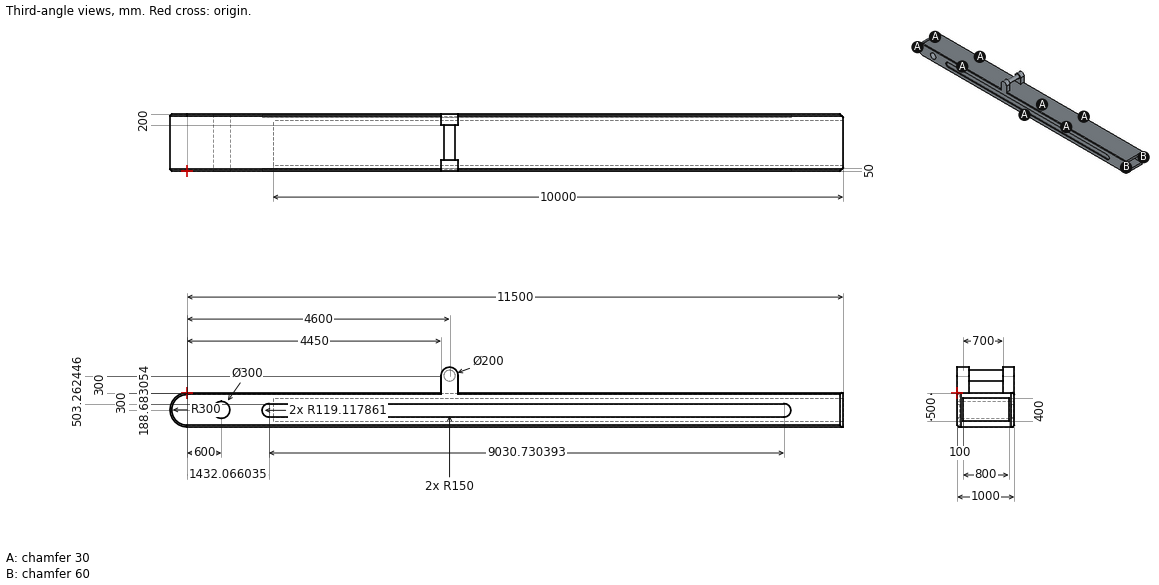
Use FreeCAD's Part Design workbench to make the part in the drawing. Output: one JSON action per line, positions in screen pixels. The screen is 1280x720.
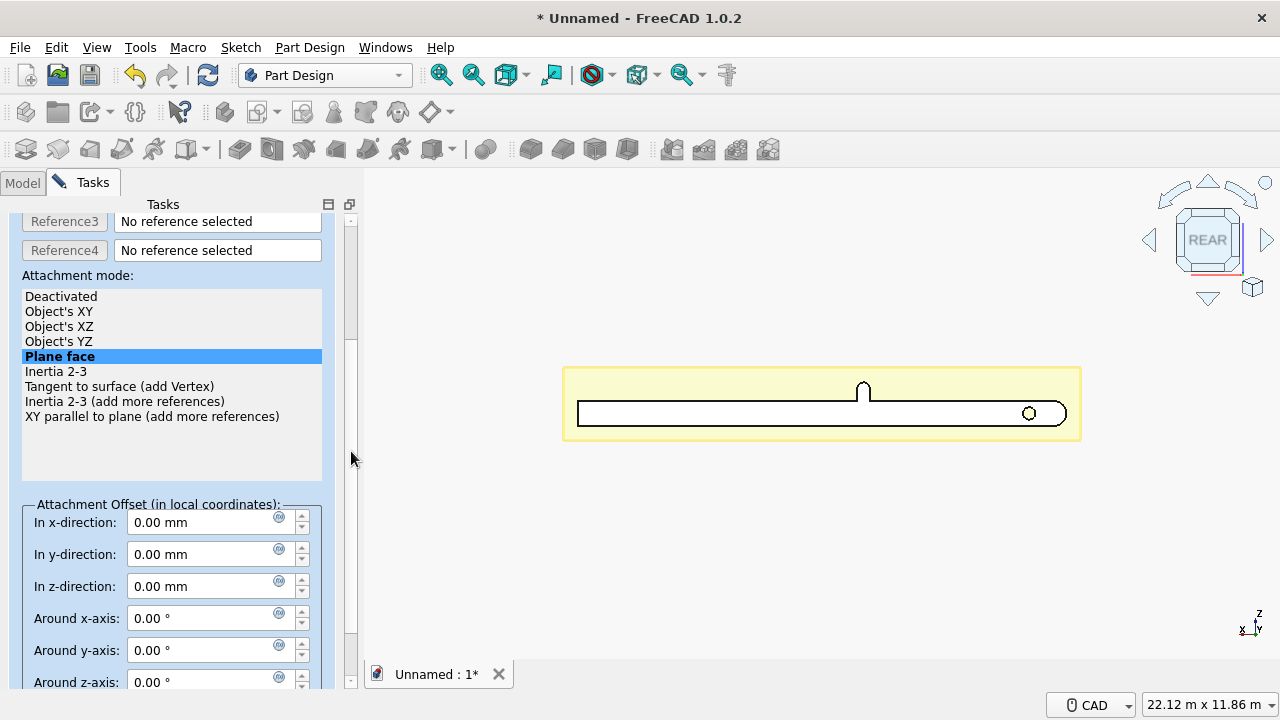
{"action": "triple_click", "coordinate": [210, 586]}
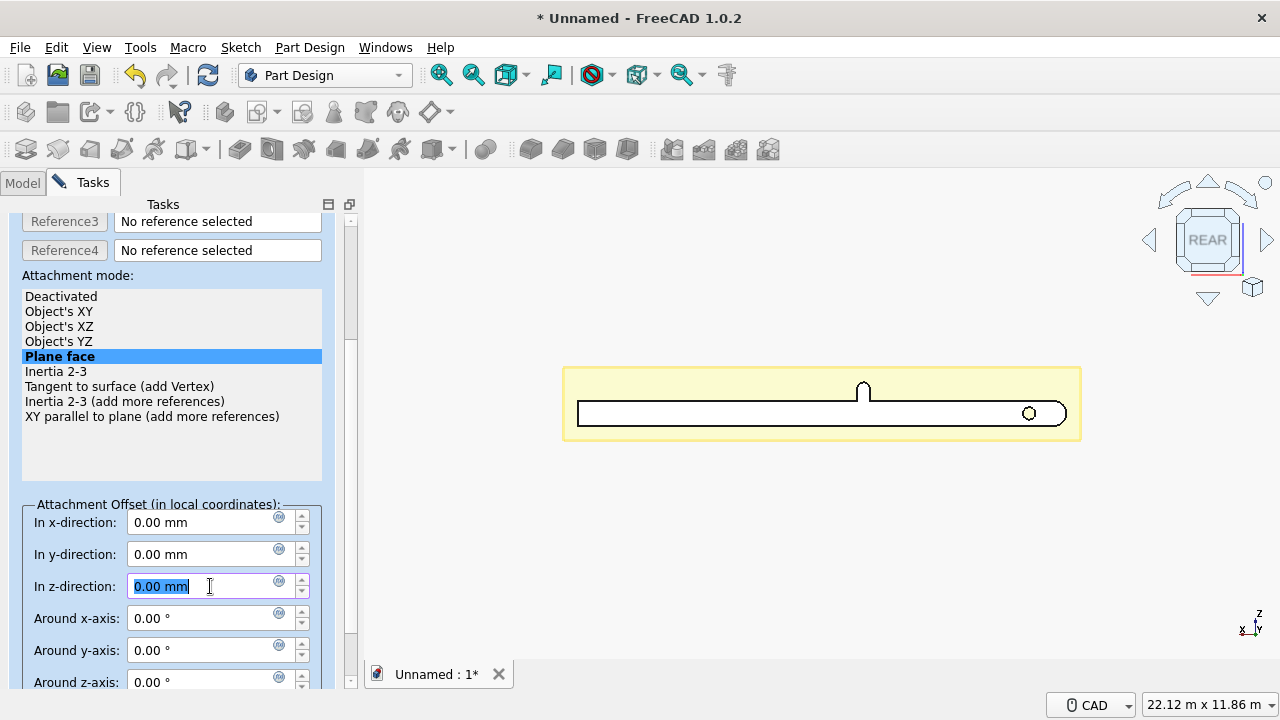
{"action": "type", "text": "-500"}
{"action": "key", "text": "Tab"}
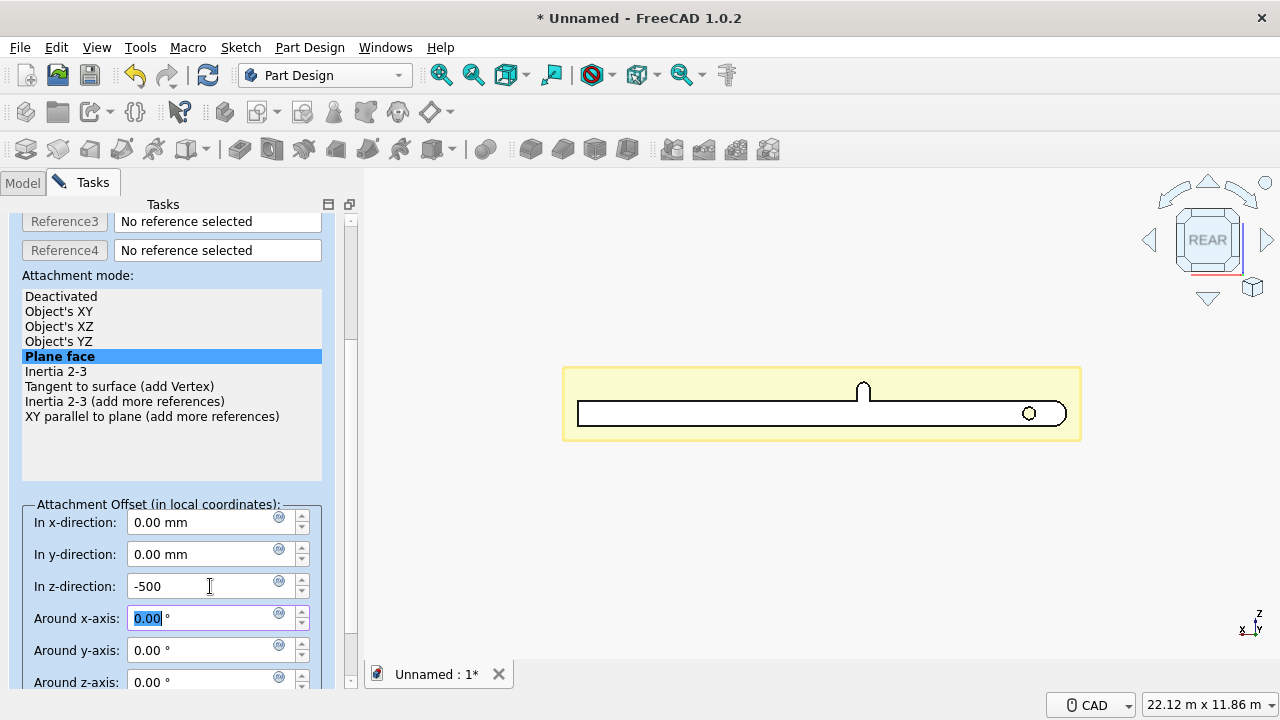
{"action": "scroll", "coordinate": [351, 451], "scroll_direction": "up", "scroll_amount": 4}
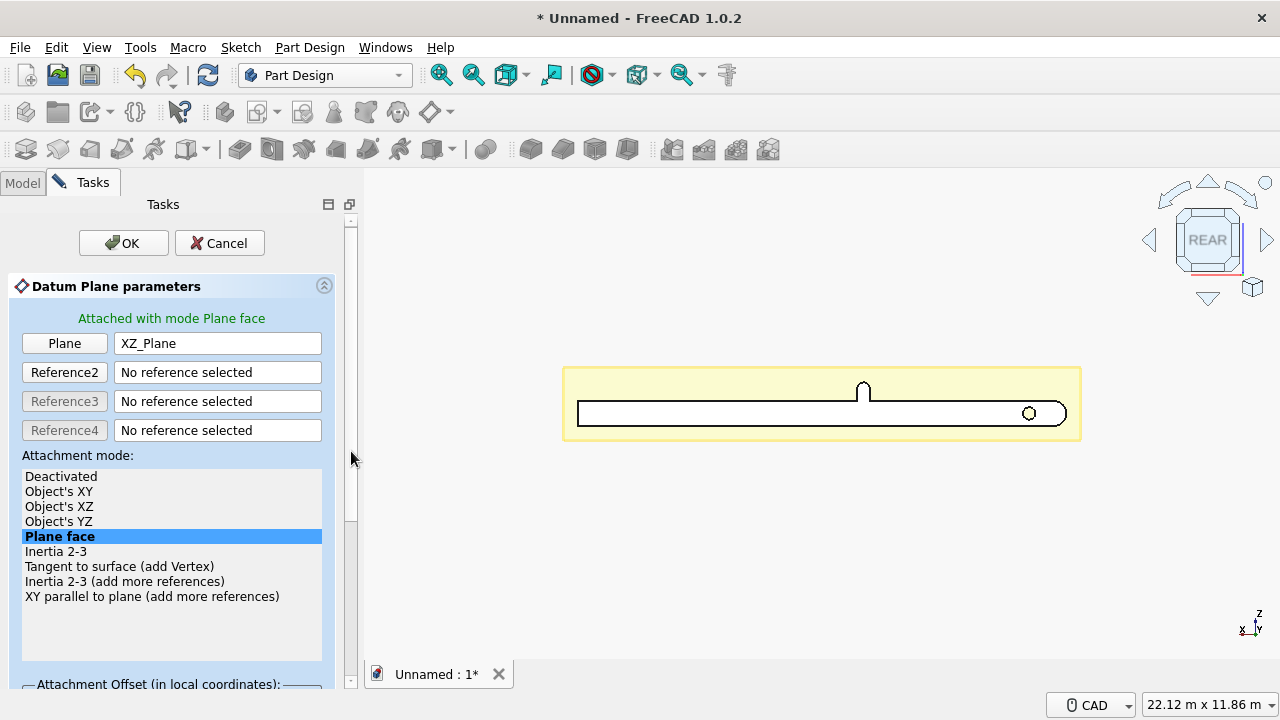
{"action": "left_click", "coordinate": [124, 243]}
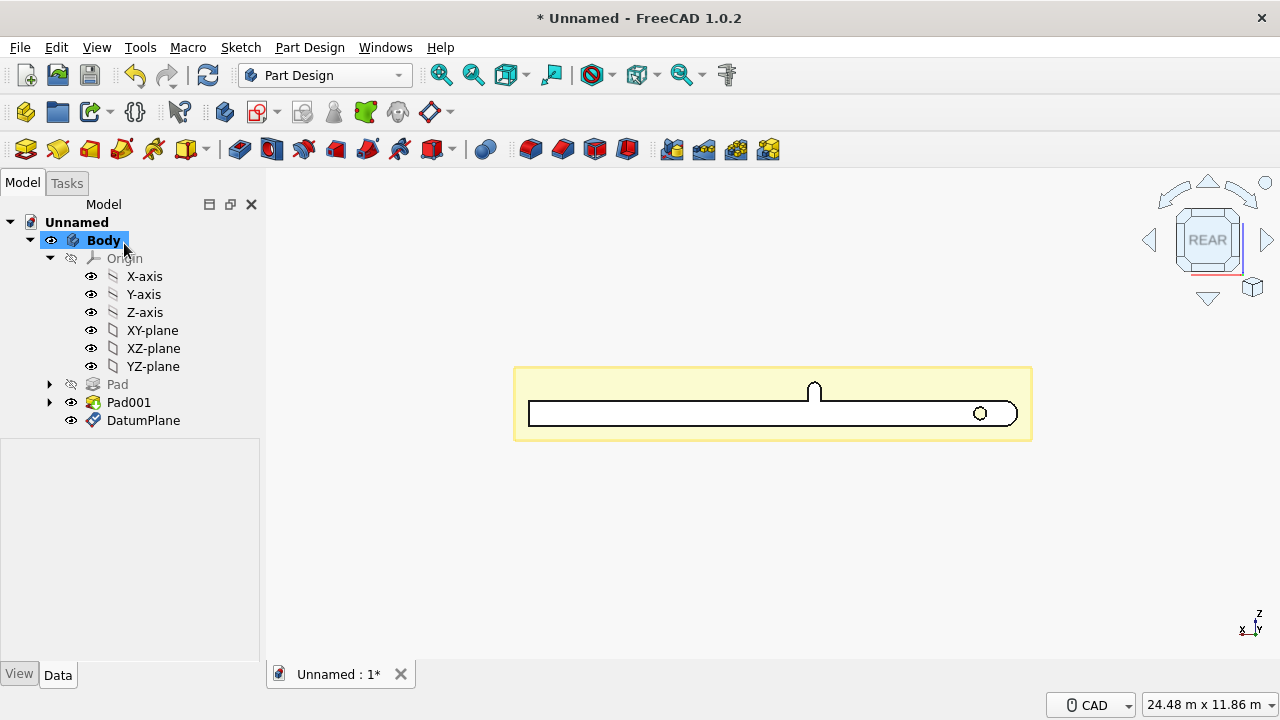
{"action": "left_click", "coordinate": [116, 402]}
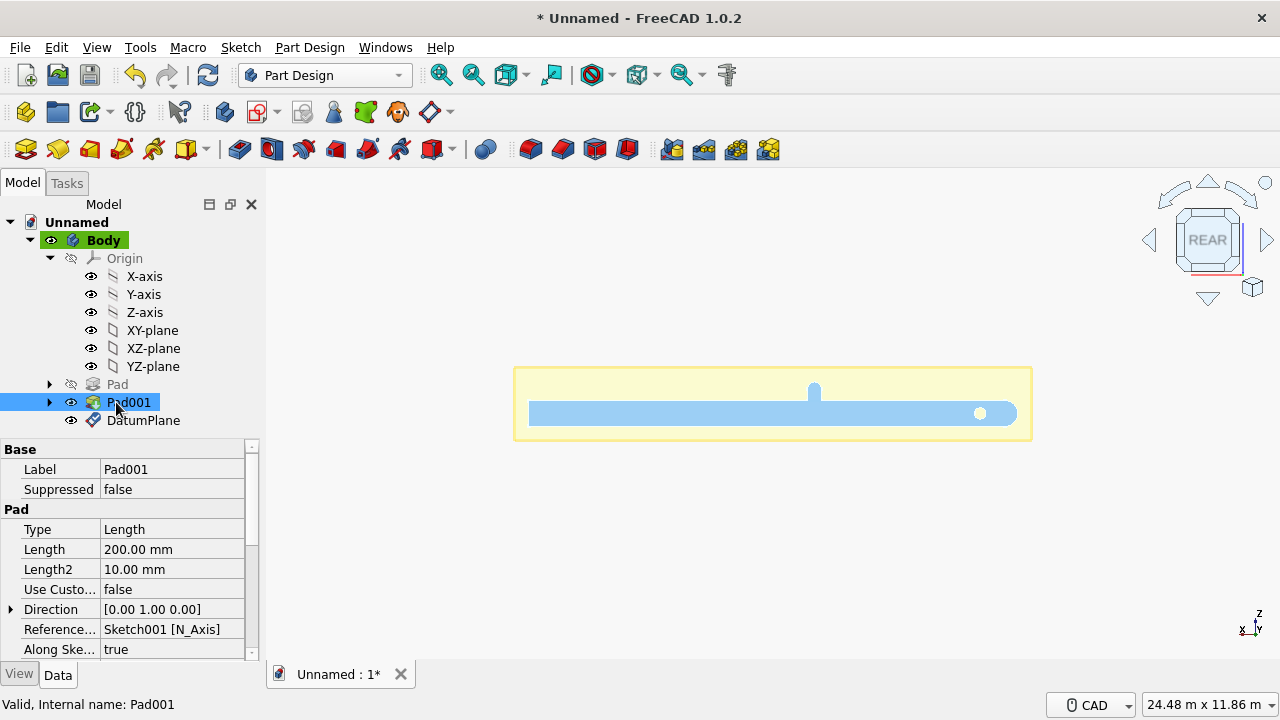
{"action": "left_click", "coordinate": [672, 150]}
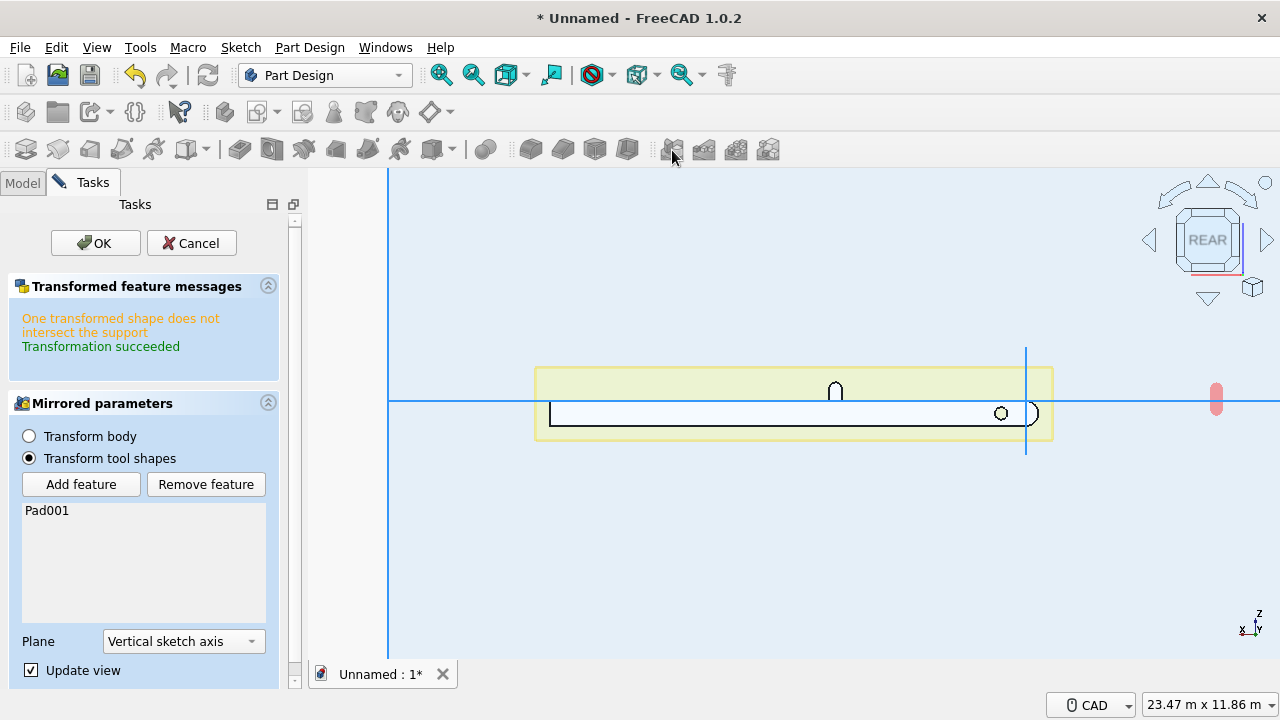
{"action": "left_click", "coordinate": [184, 642]}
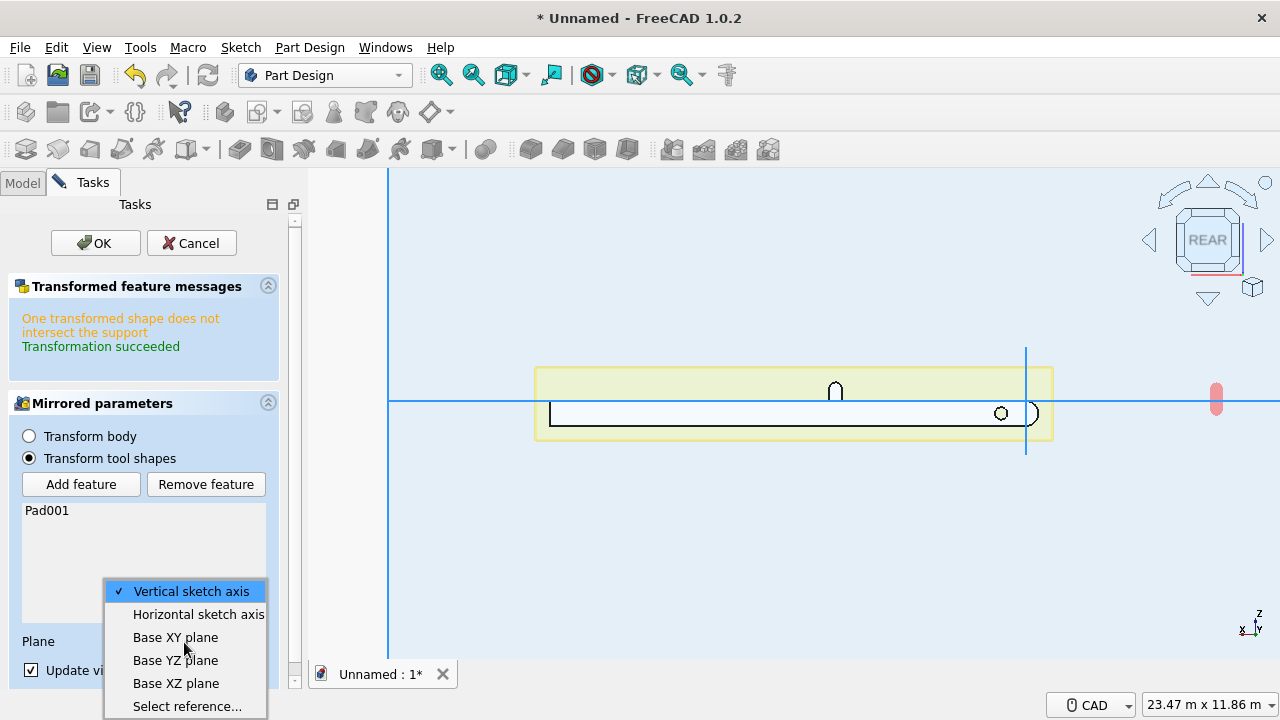
{"action": "left_click", "coordinate": [184, 706]}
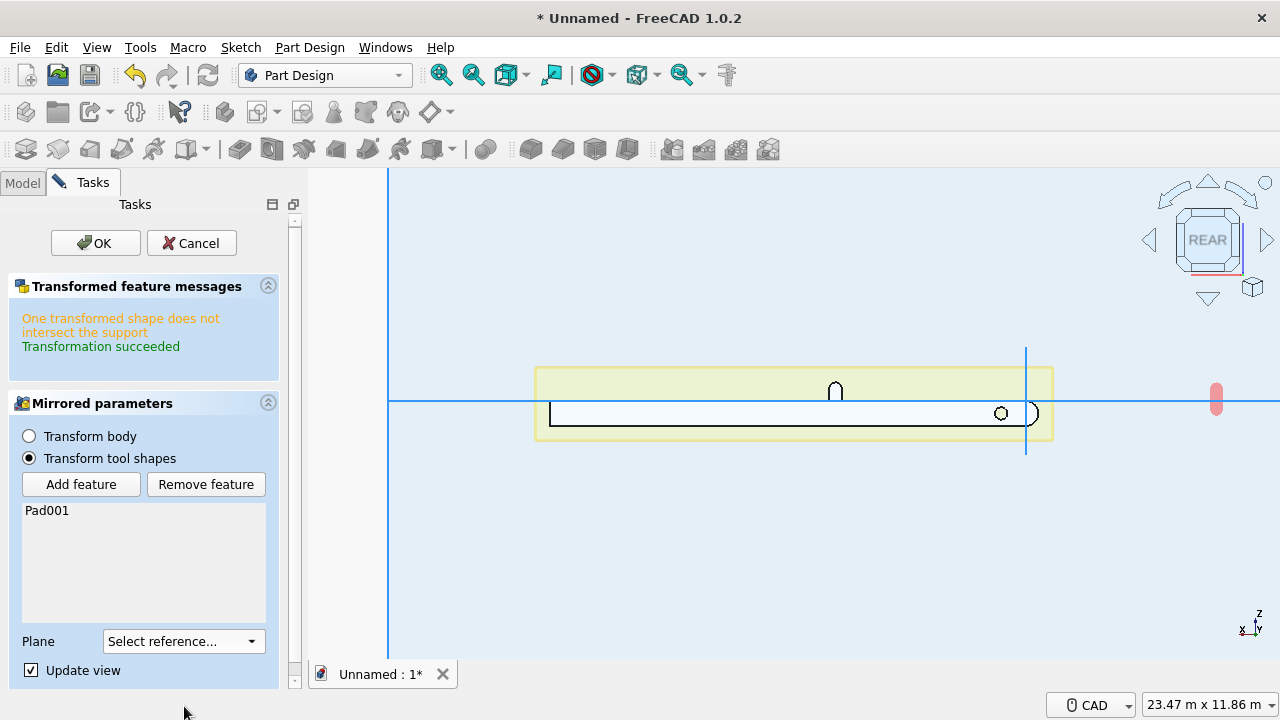
{"action": "left_click", "coordinate": [23, 182]}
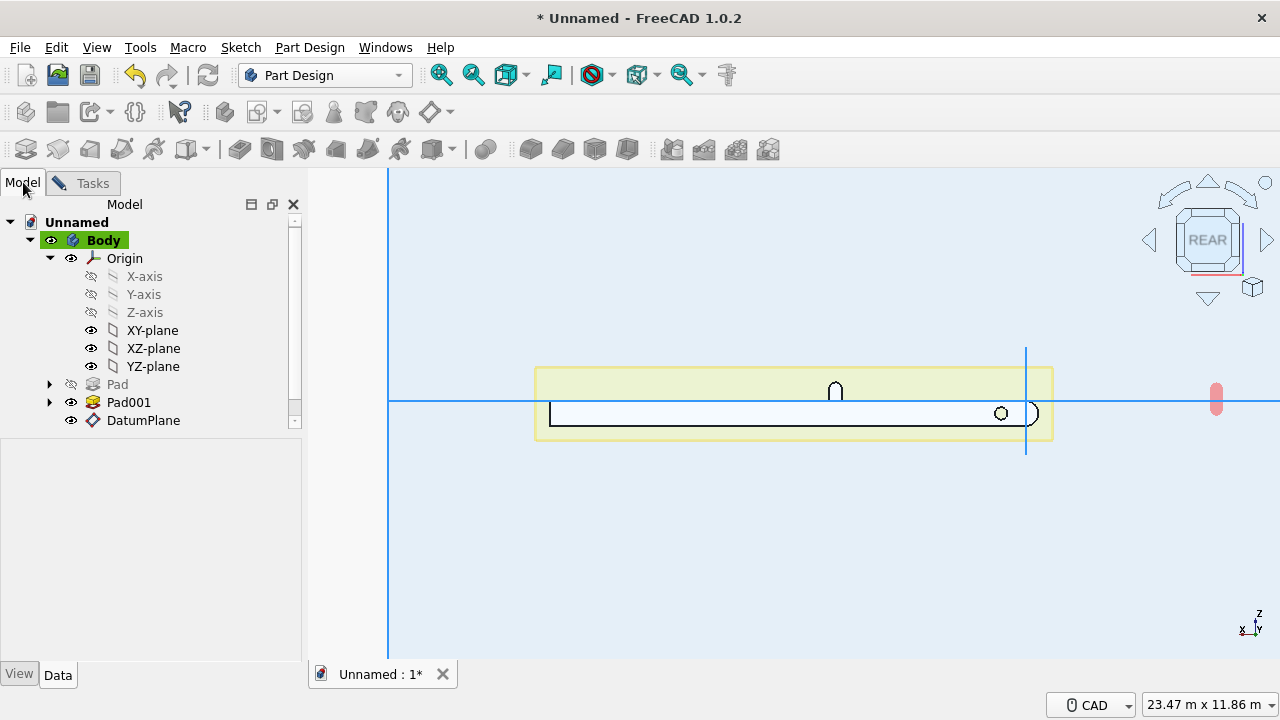
{"action": "left_click", "coordinate": [116, 420]}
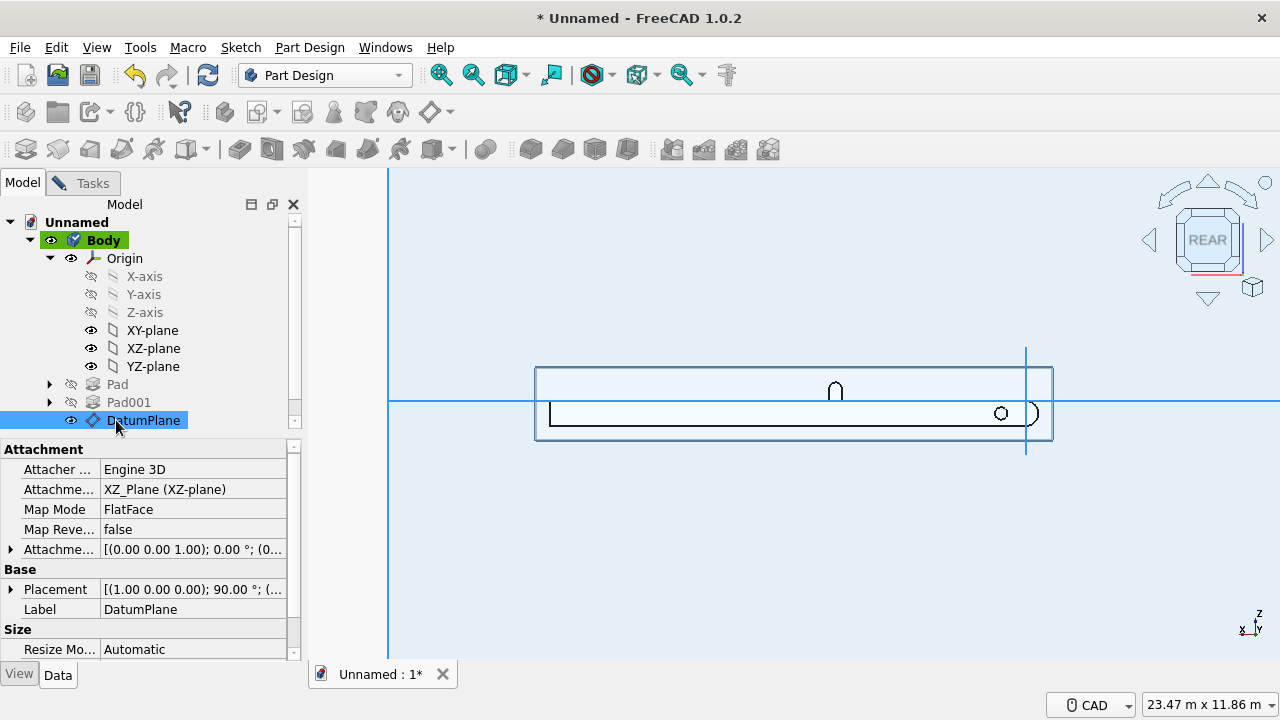
{"action": "left_click", "coordinate": [84, 182]}